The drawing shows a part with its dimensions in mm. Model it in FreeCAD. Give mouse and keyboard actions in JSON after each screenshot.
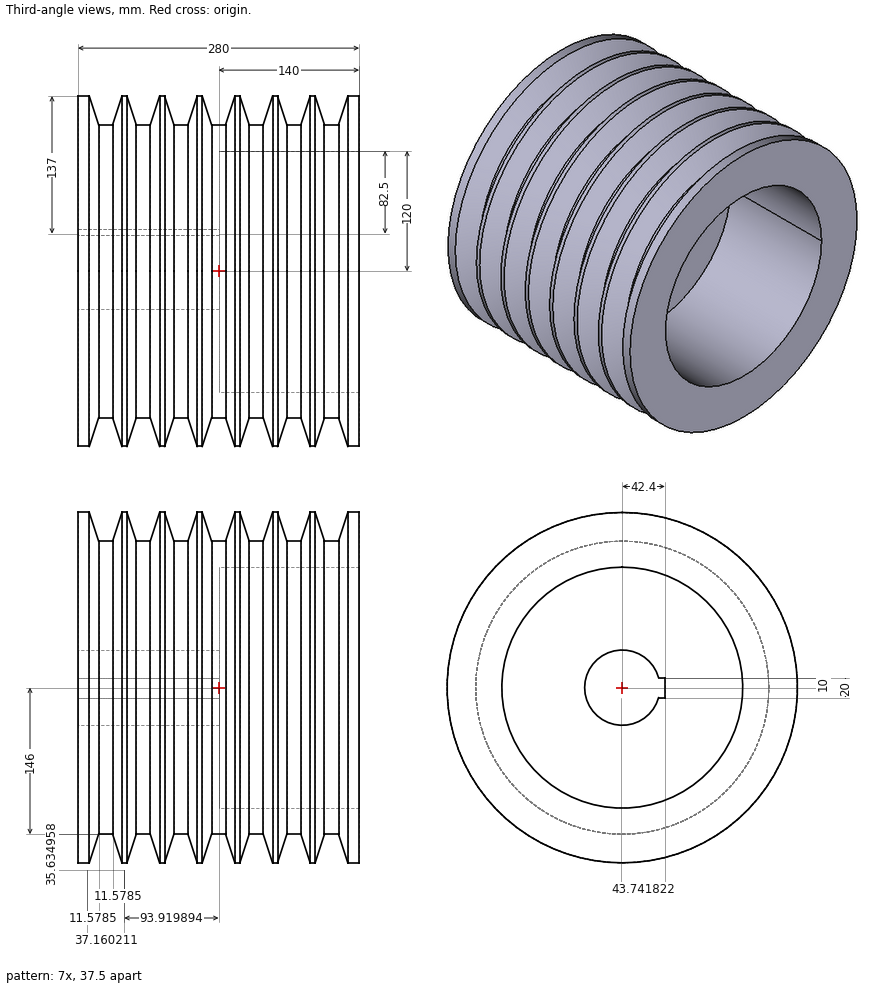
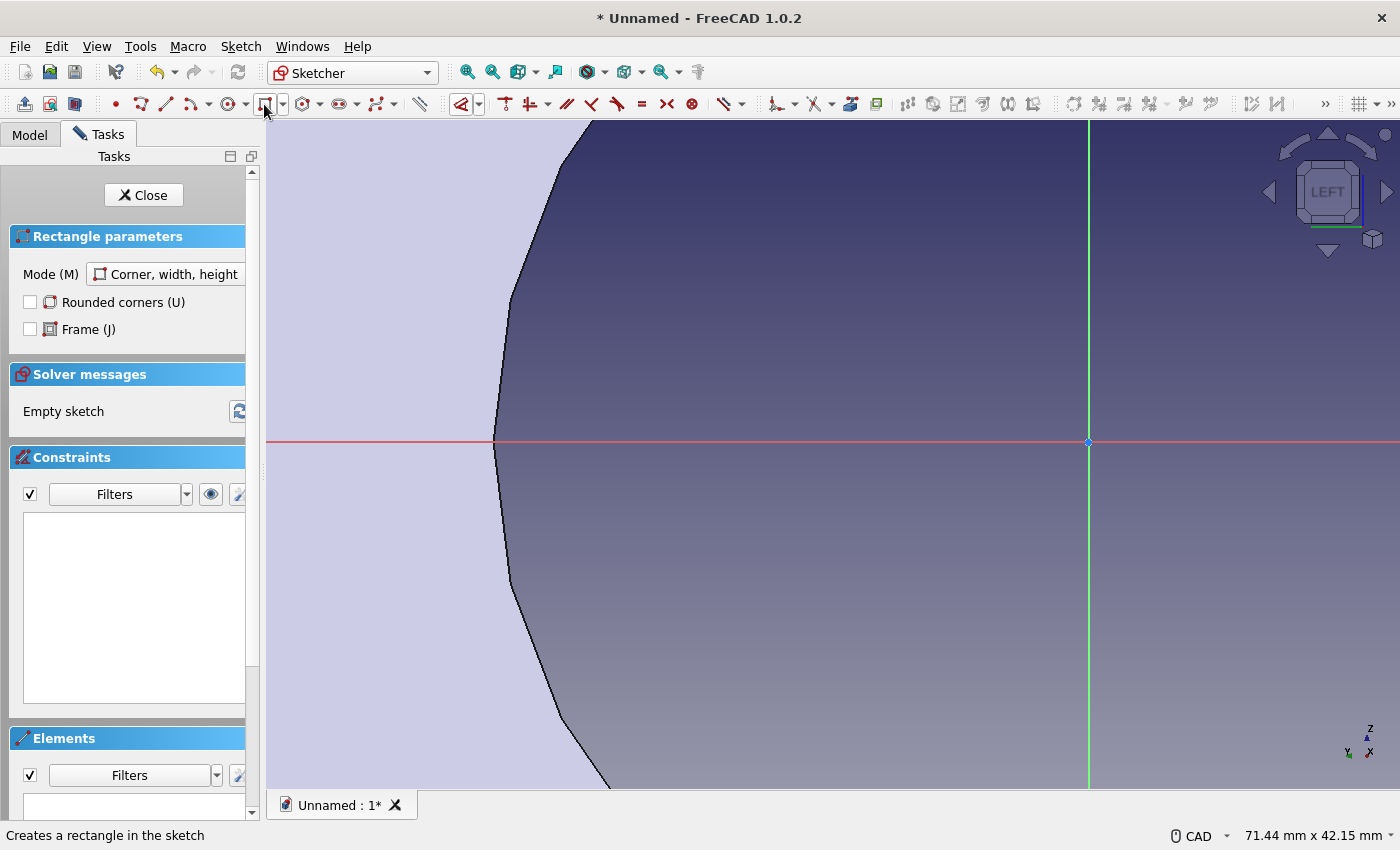
{"action": "left_click", "coordinate": [416, 283]}
{"action": "left_click", "coordinate": [1110, 601]}
{"action": "key", "text": "Escape"}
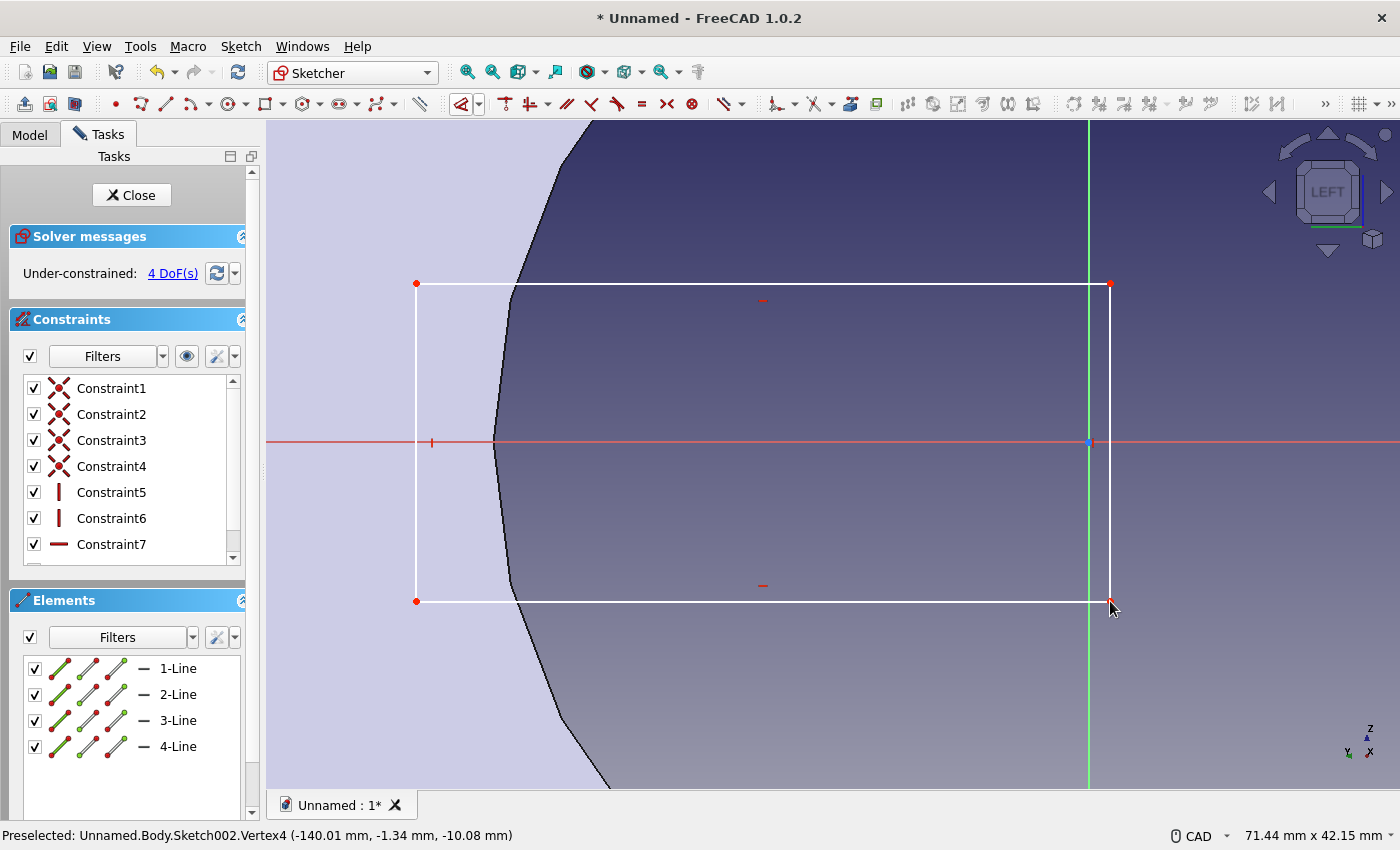
{"action": "left_click", "coordinate": [416, 379]}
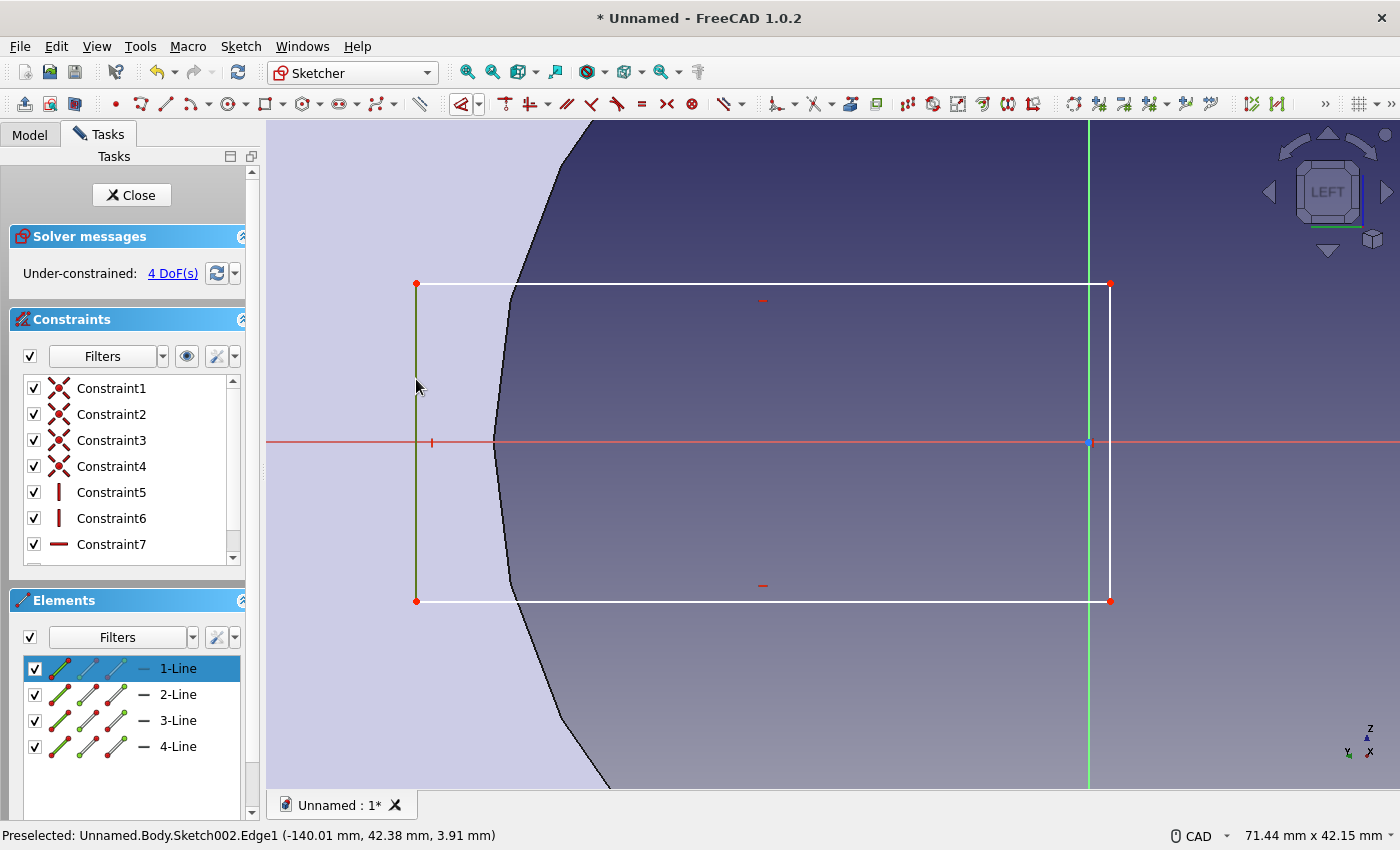
{"action": "left_click", "coordinate": [478, 104]}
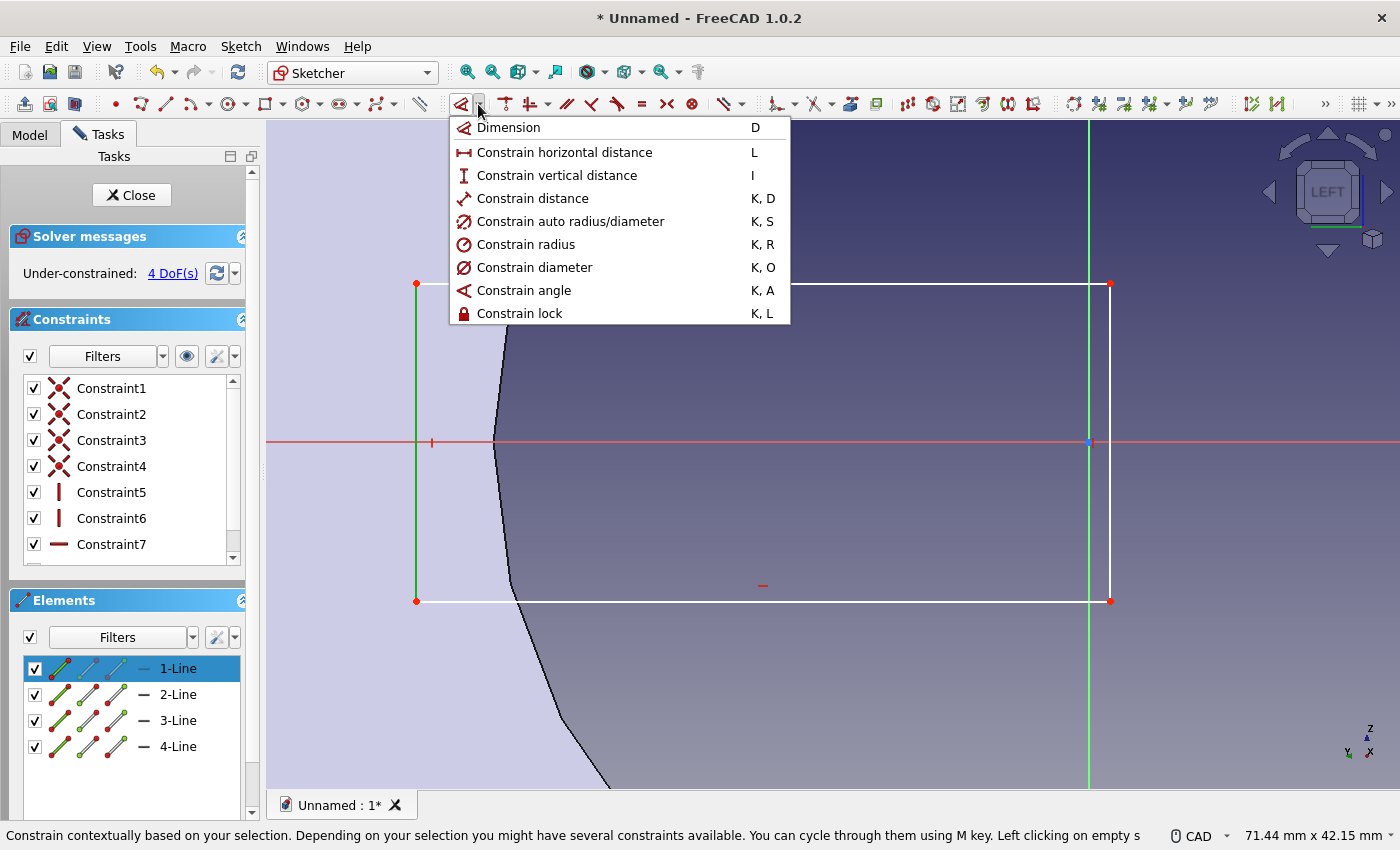
{"action": "left_click", "coordinate": [620, 176]}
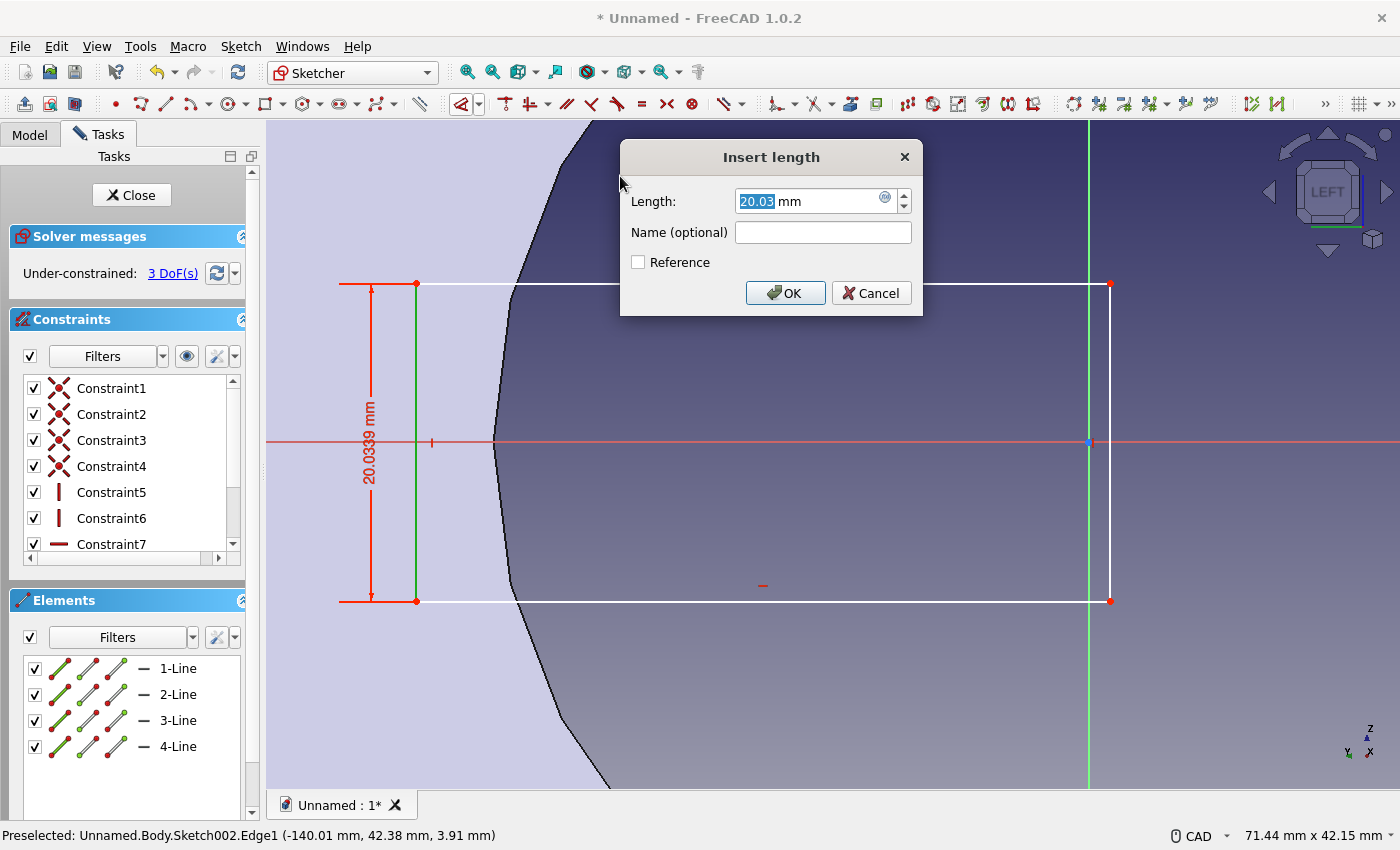
{"action": "type", "text": "20"}
{"action": "key", "text": "Return"}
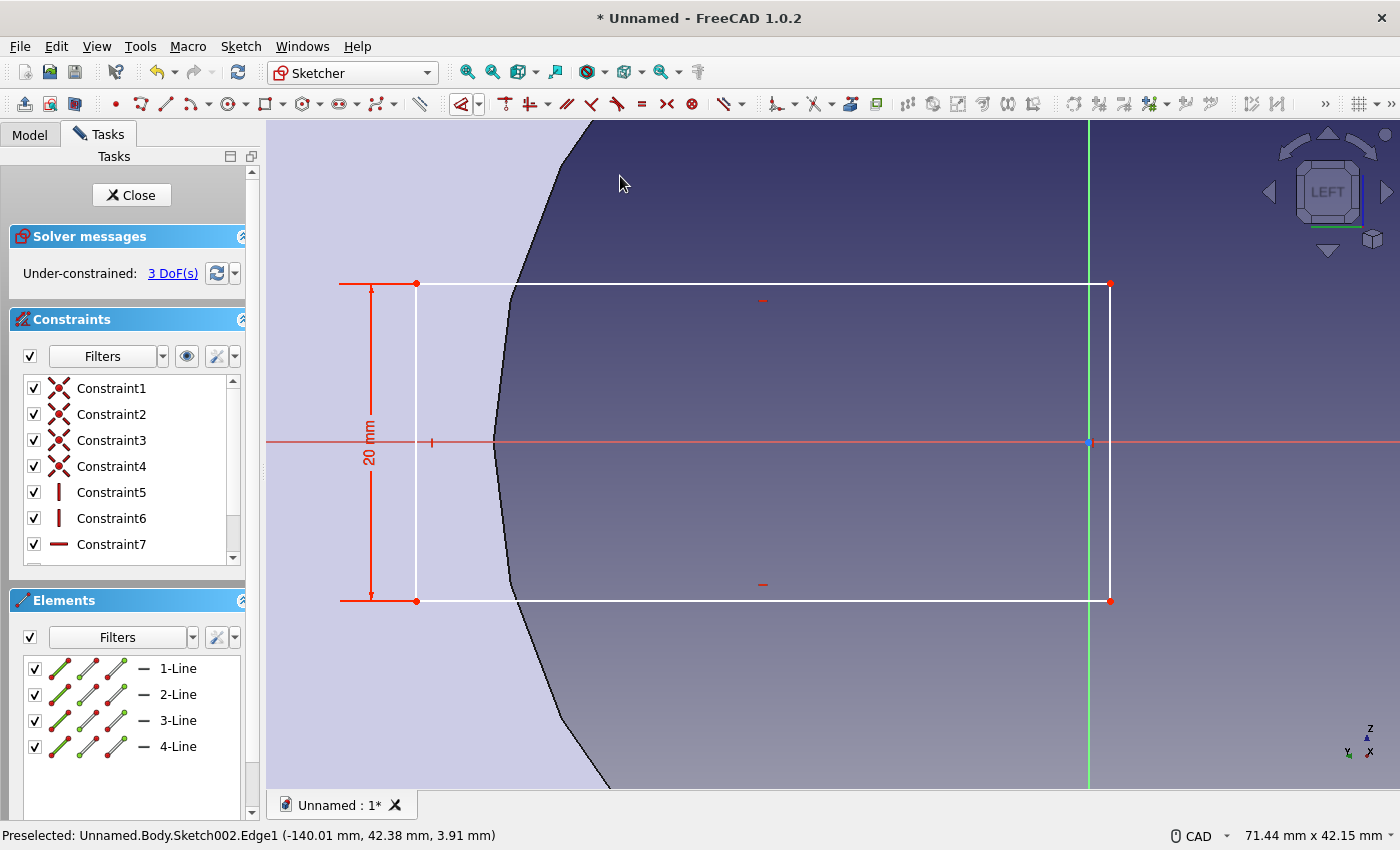
{"action": "left_click", "coordinate": [416, 284]}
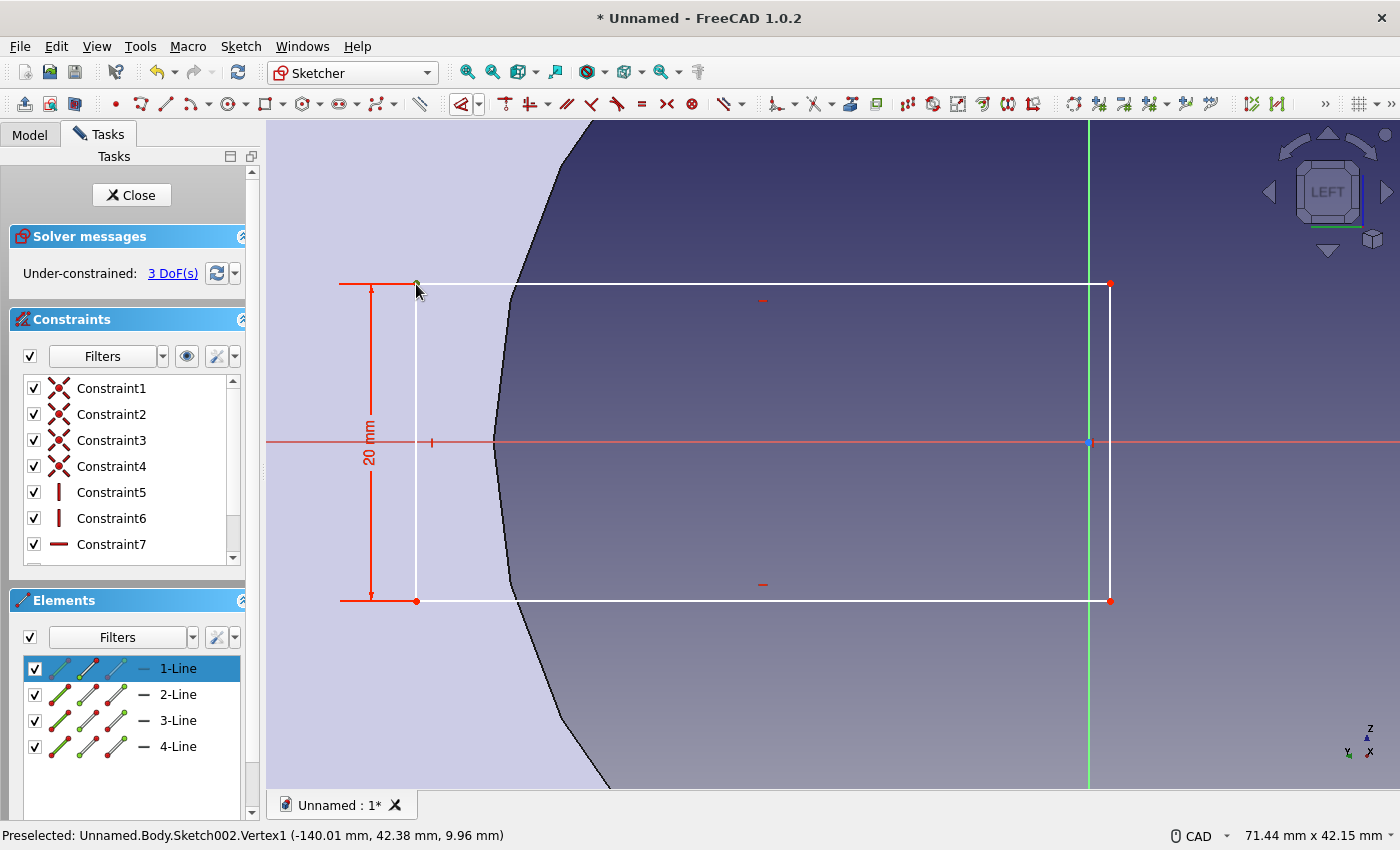
{"action": "left_click", "coordinate": [478, 104]}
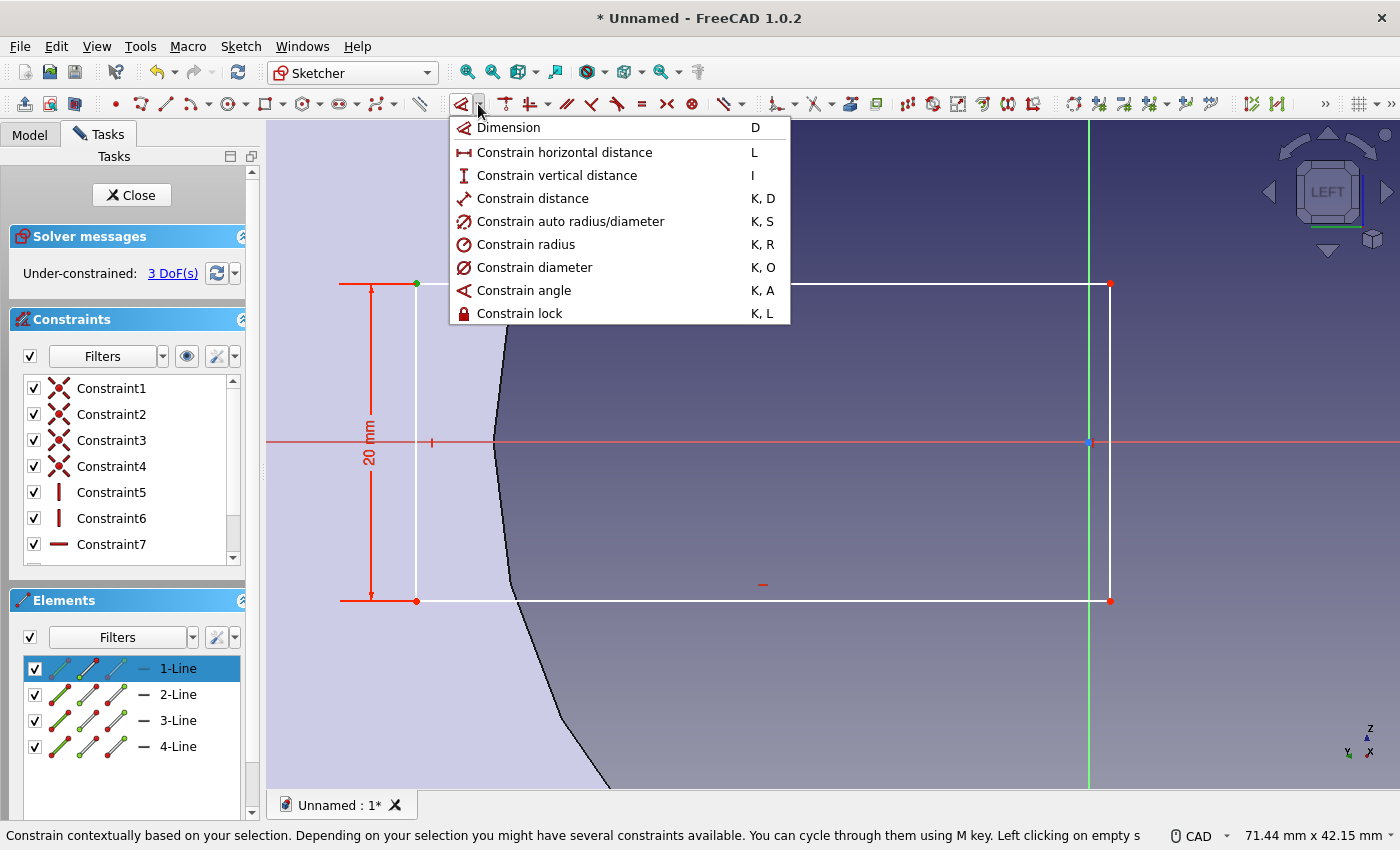
{"action": "left_click", "coordinate": [620, 176]}